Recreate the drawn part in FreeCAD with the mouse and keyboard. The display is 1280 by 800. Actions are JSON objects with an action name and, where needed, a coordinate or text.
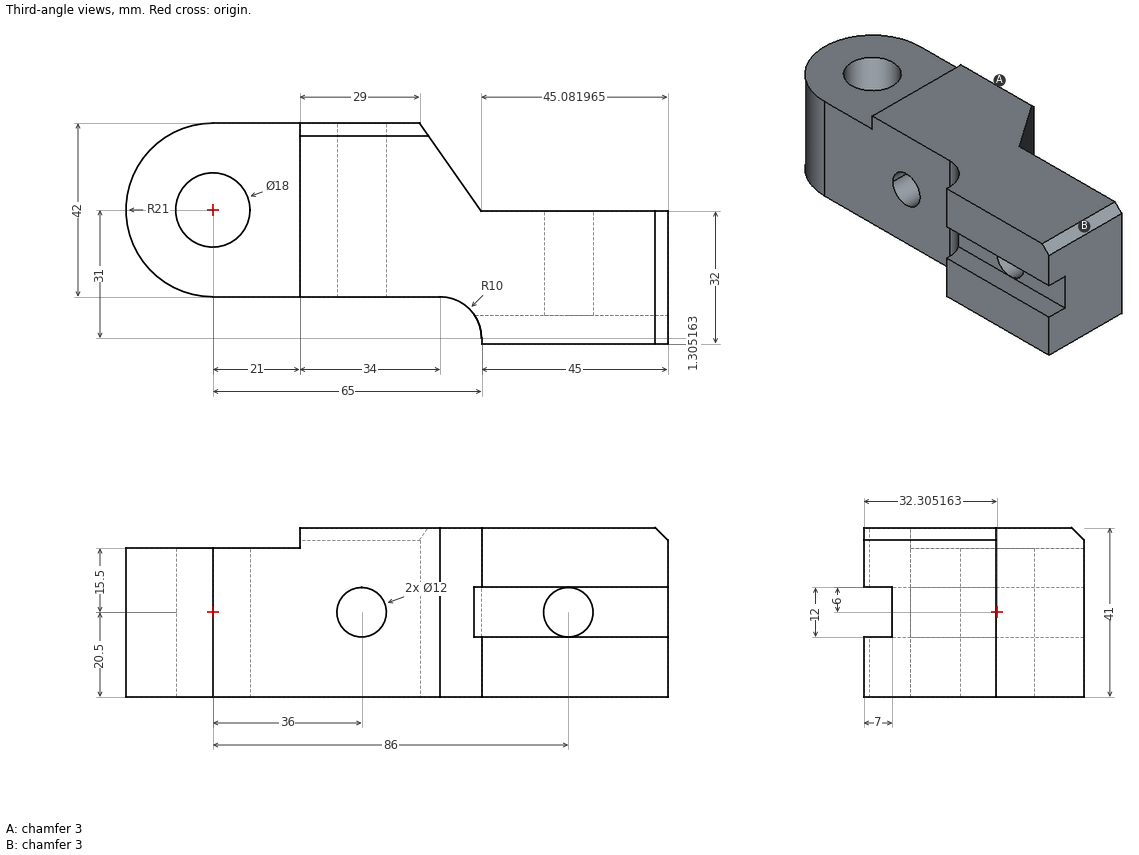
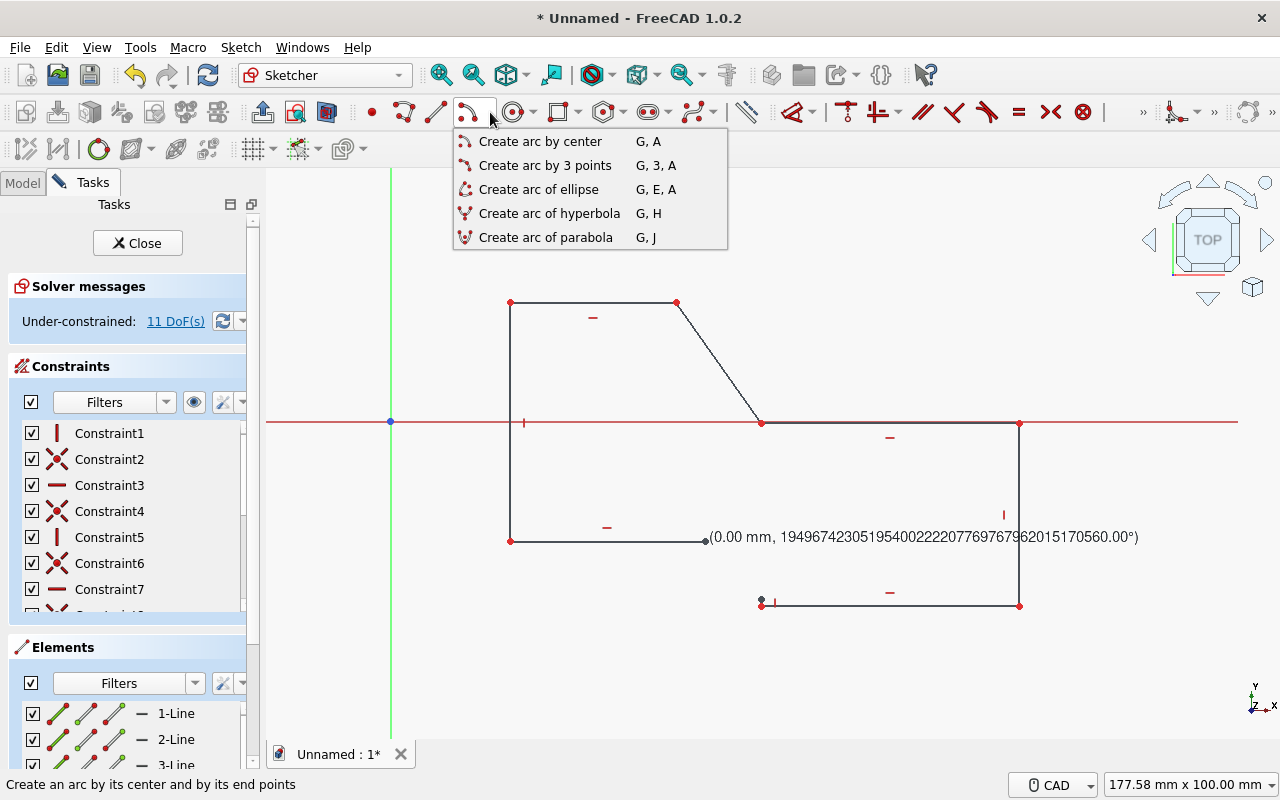
{"action": "left_click", "coordinate": [590, 165]}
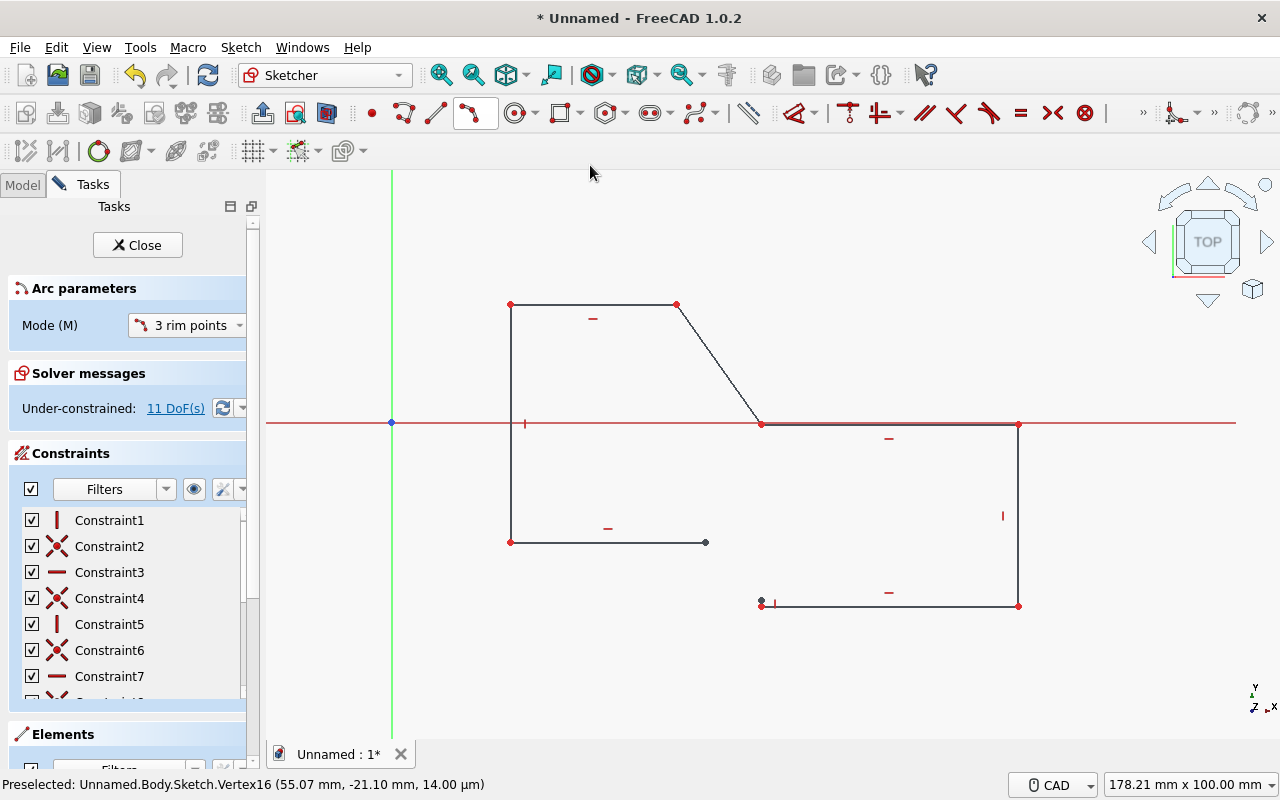
{"action": "left_click", "coordinate": [705, 543]}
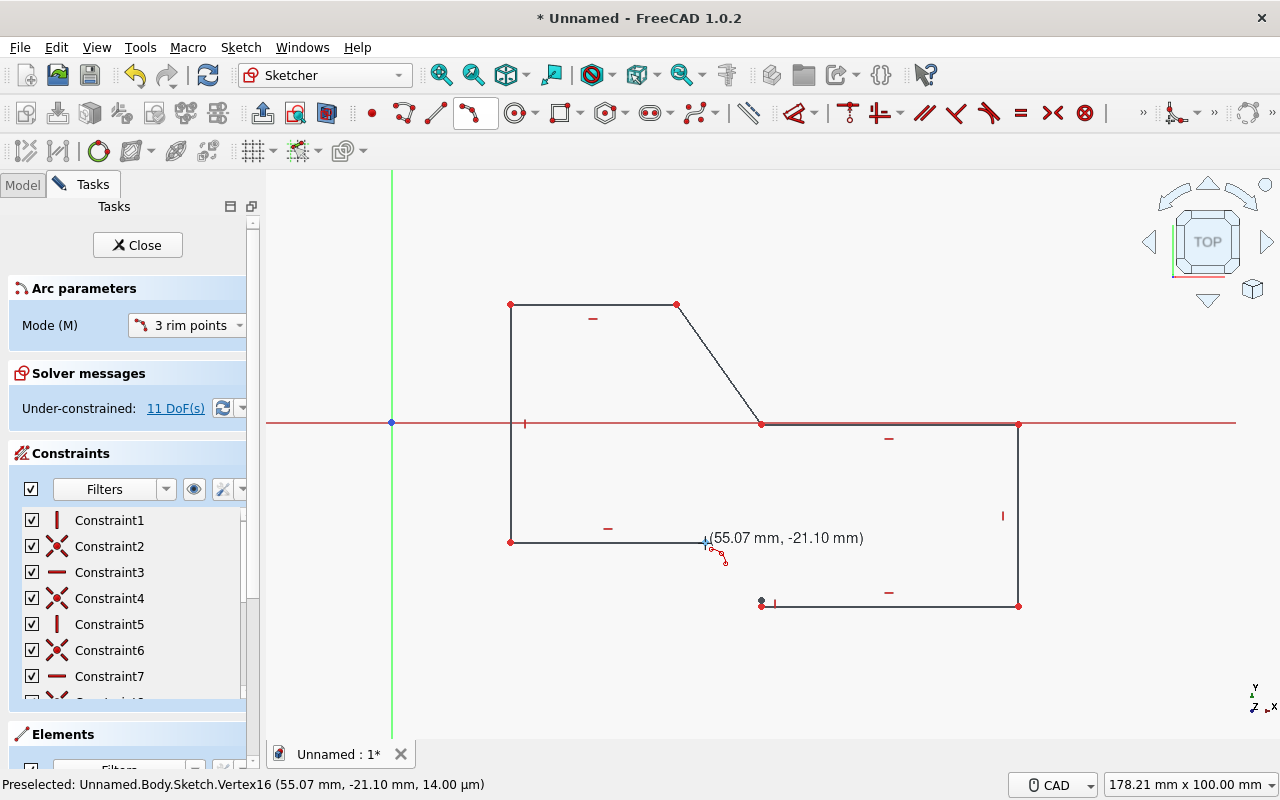
{"action": "scroll", "coordinate": [762, 599], "scroll_direction": "up", "scroll_amount": 8}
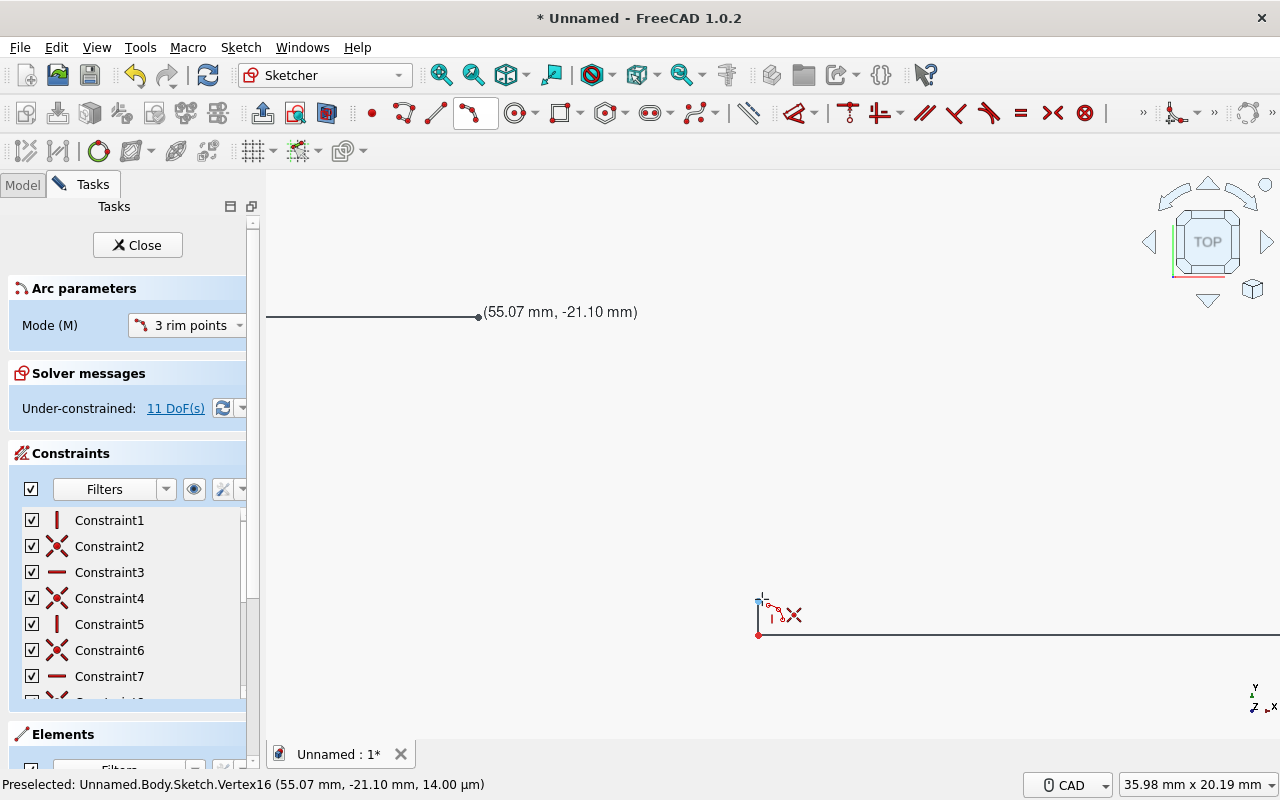
{"action": "left_click", "coordinate": [758, 601]}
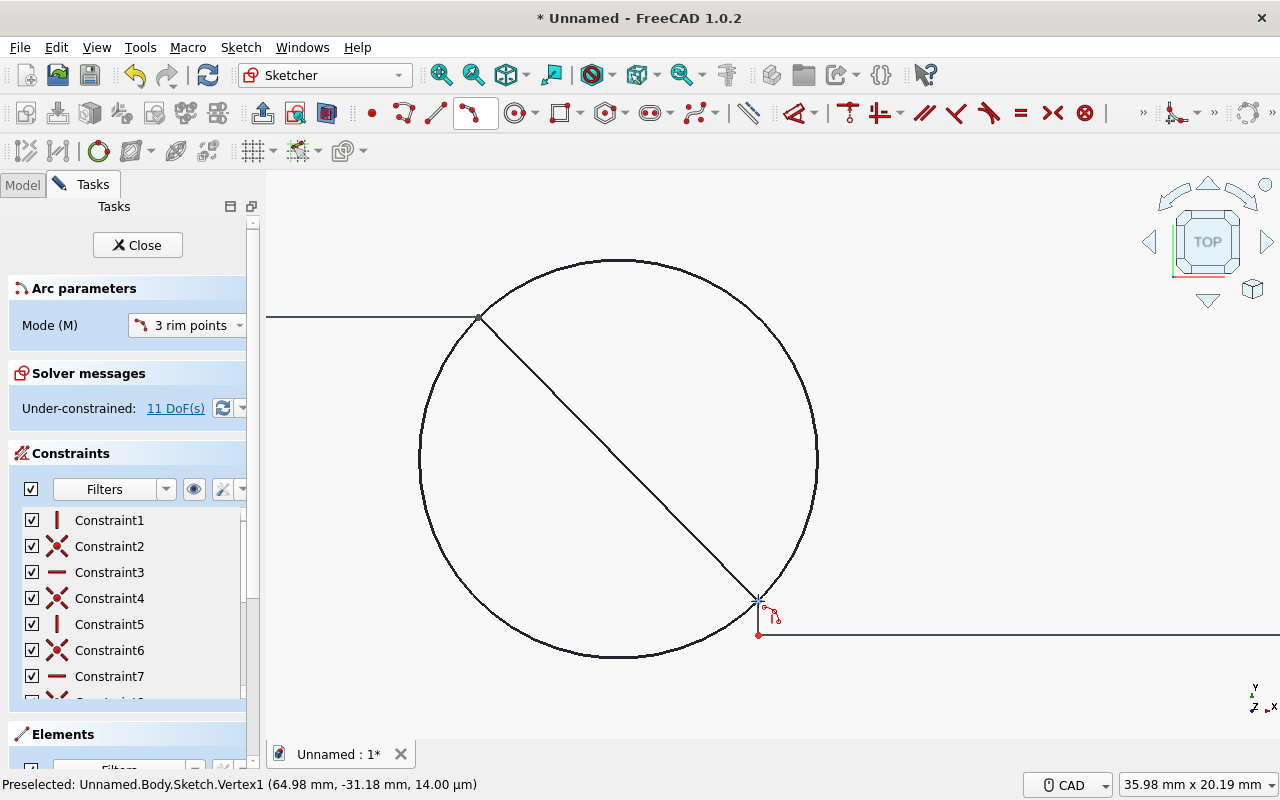
{"action": "scroll", "coordinate": [762, 599], "scroll_direction": "down", "scroll_amount": 8}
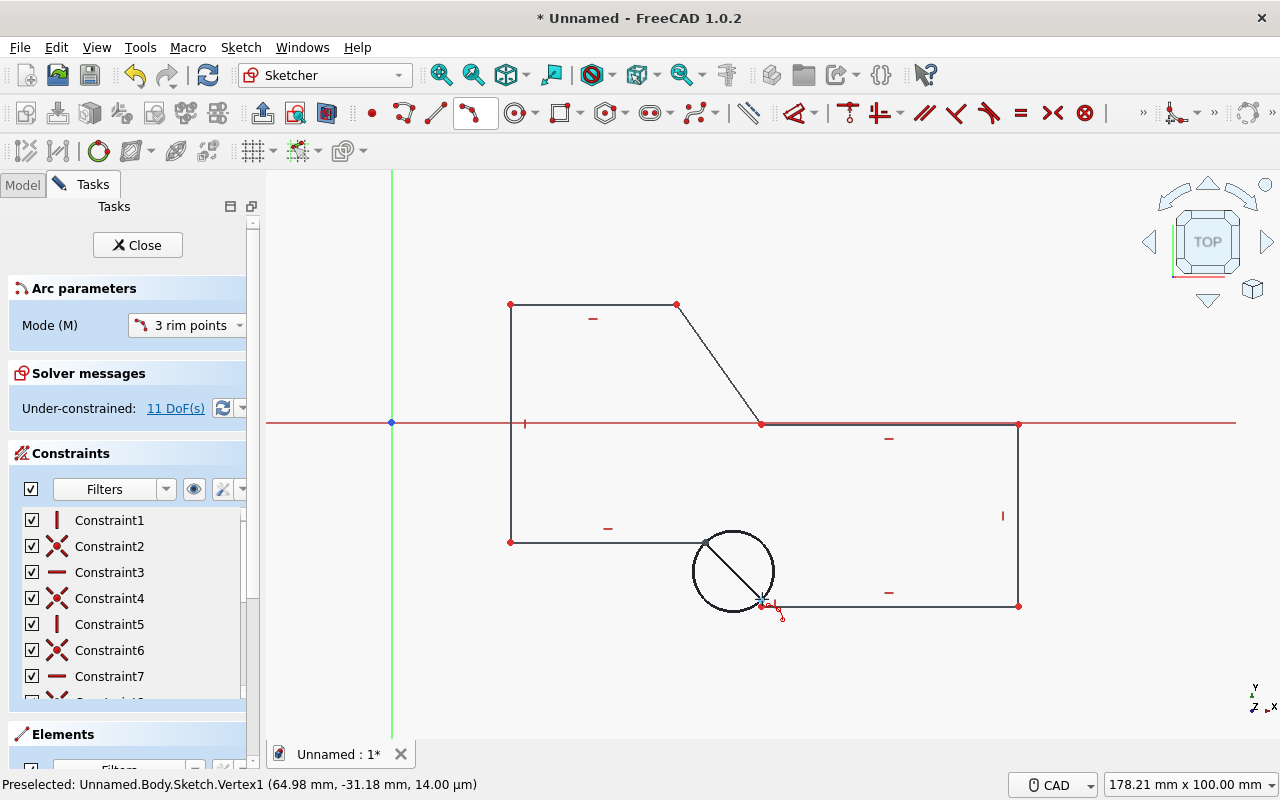
{"action": "left_click", "coordinate": [745, 559]}
{"action": "key", "text": "Escape"}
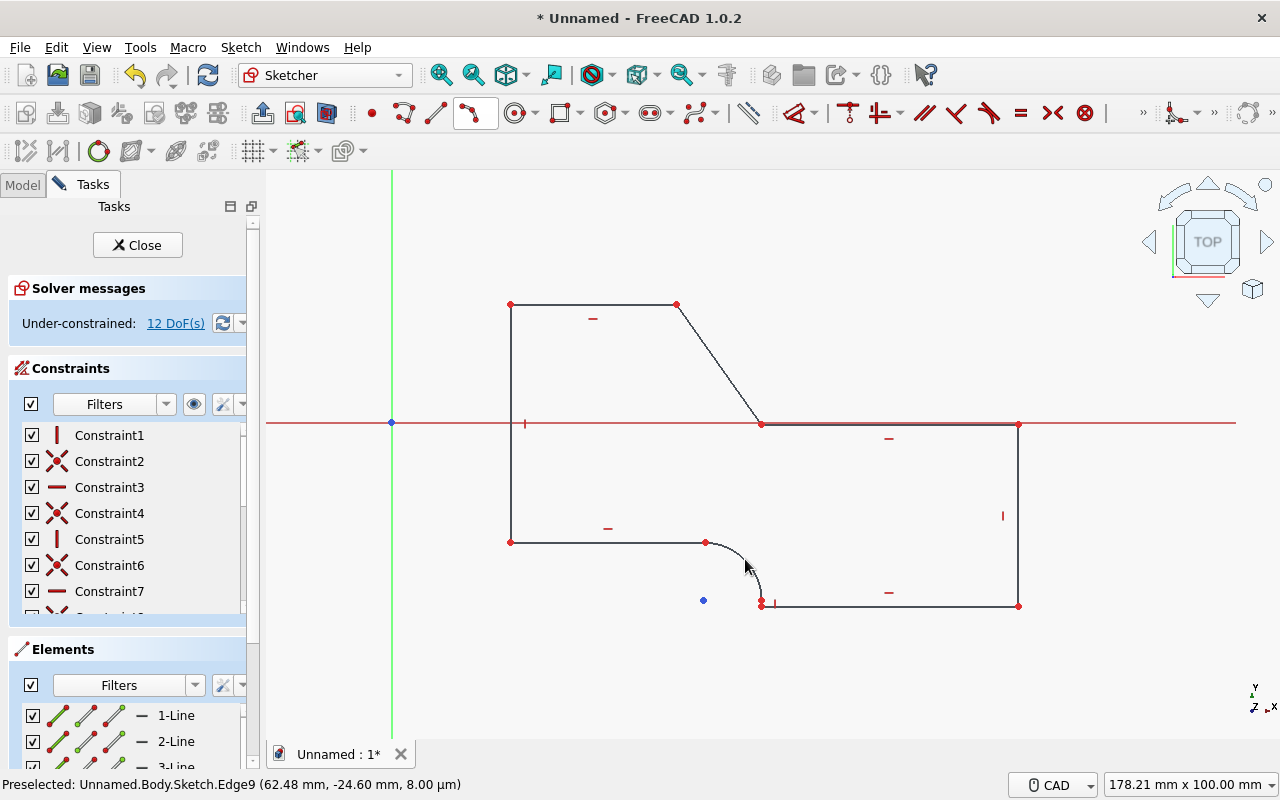
{"action": "scroll", "coordinate": [762, 603], "scroll_direction": "up", "scroll_amount": 7}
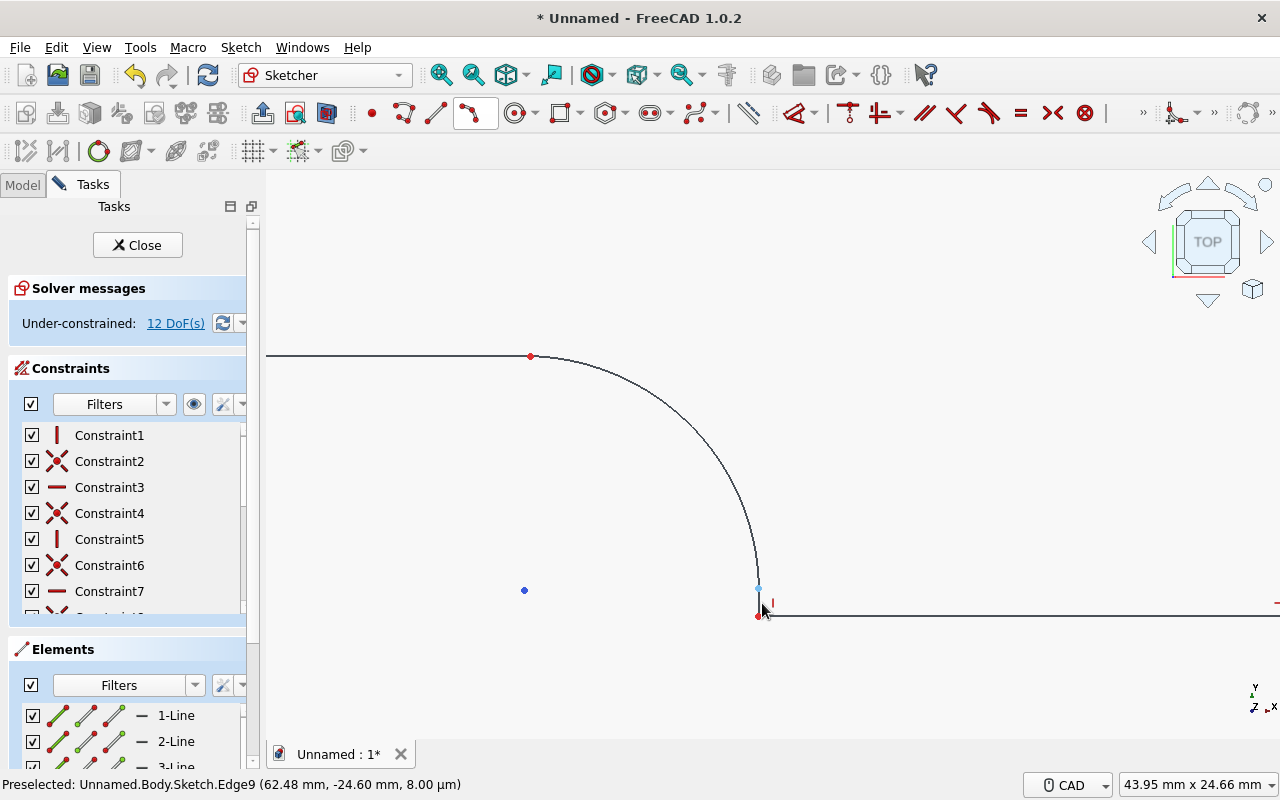
{"action": "left_click", "coordinate": [759, 603]}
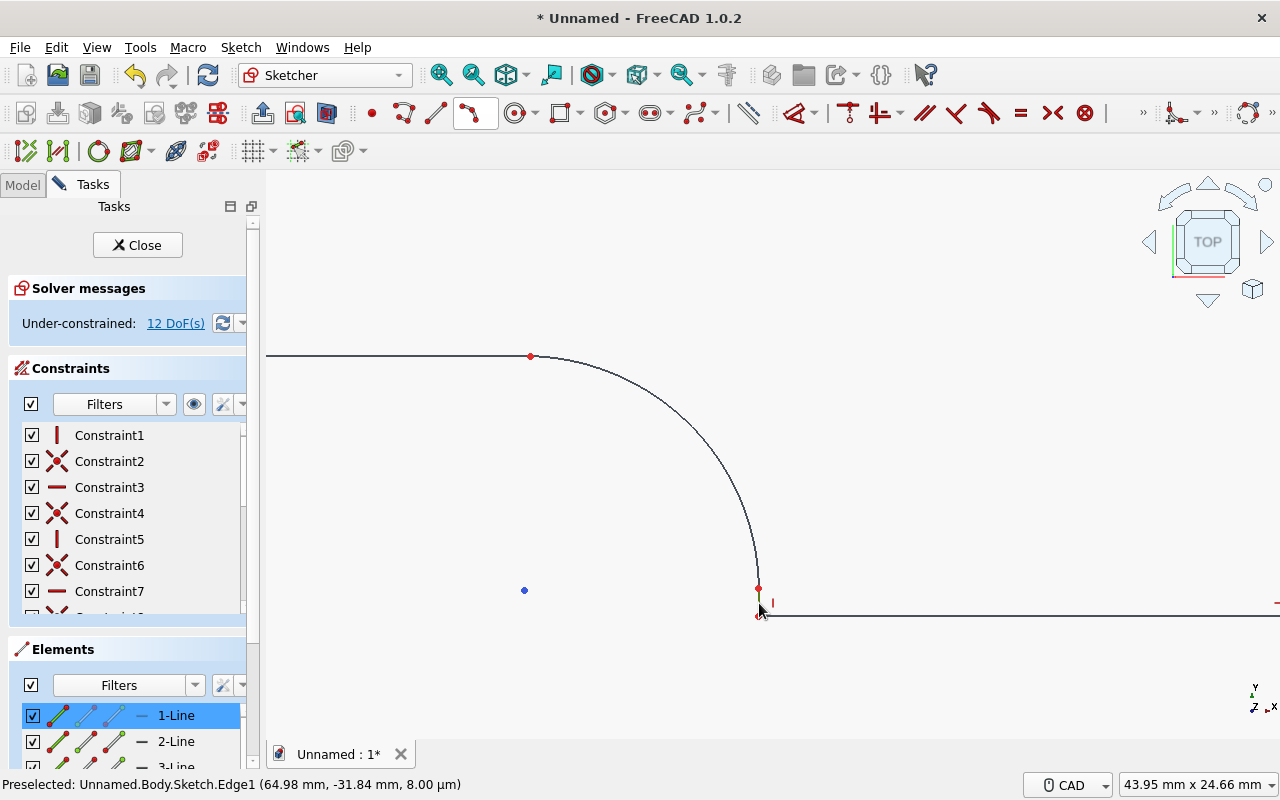
{"action": "scroll", "coordinate": [762, 603], "scroll_direction": "down", "scroll_amount": 7}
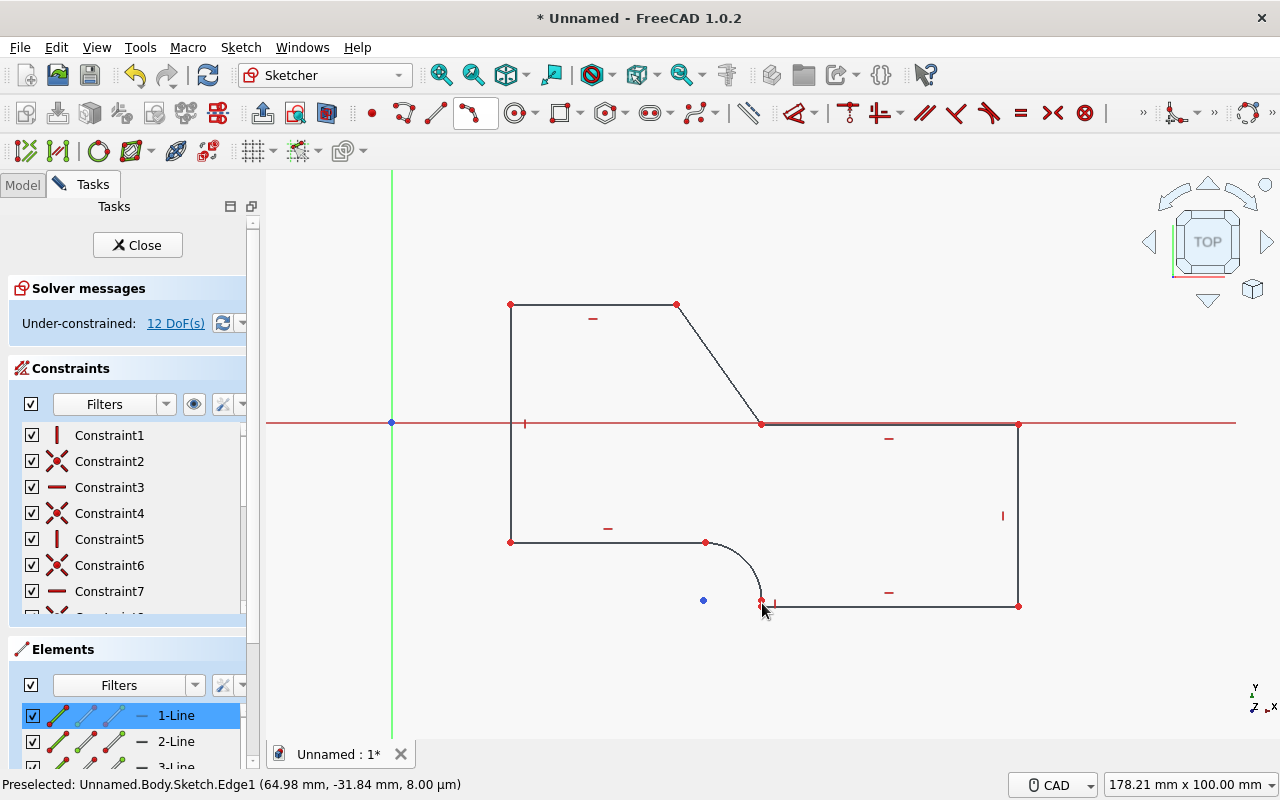
{"action": "left_click", "coordinate": [755, 574]}